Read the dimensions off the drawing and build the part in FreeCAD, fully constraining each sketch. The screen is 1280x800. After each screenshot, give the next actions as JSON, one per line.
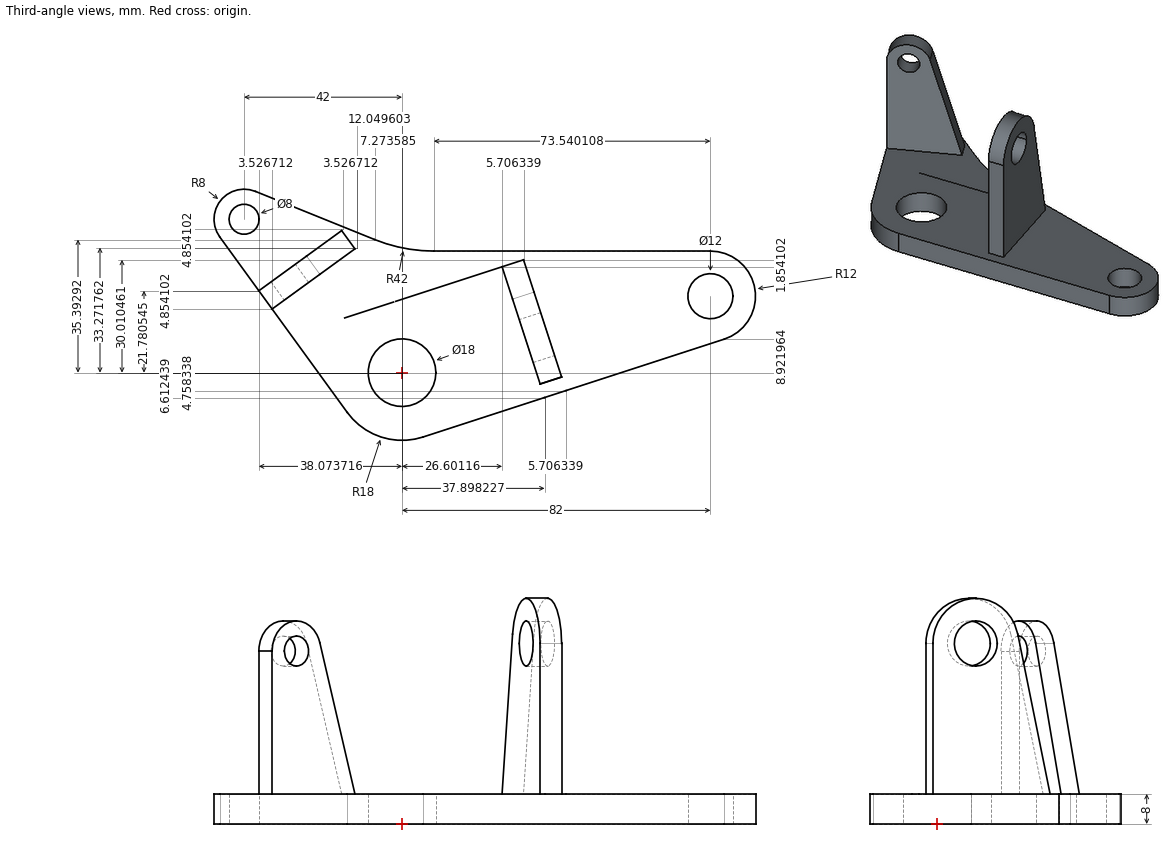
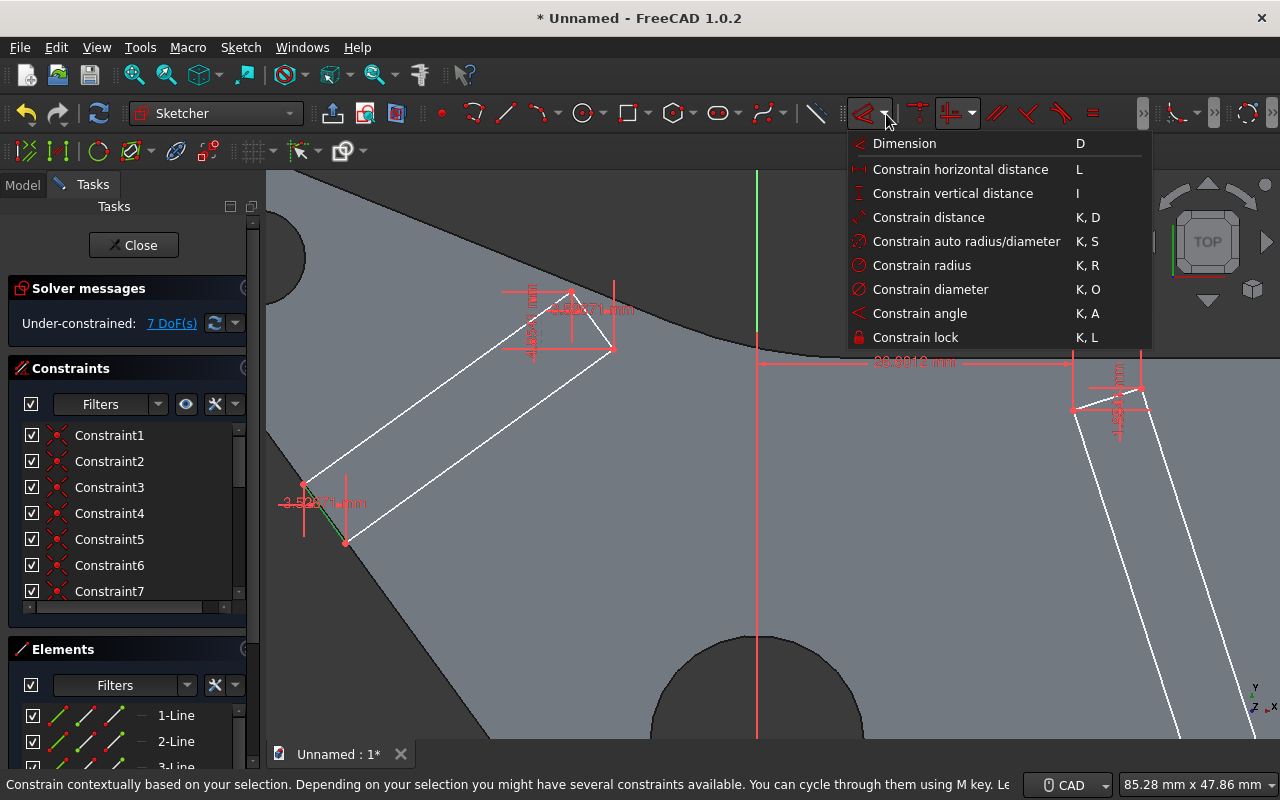
{"action": "left_click", "coordinate": [1000, 193]}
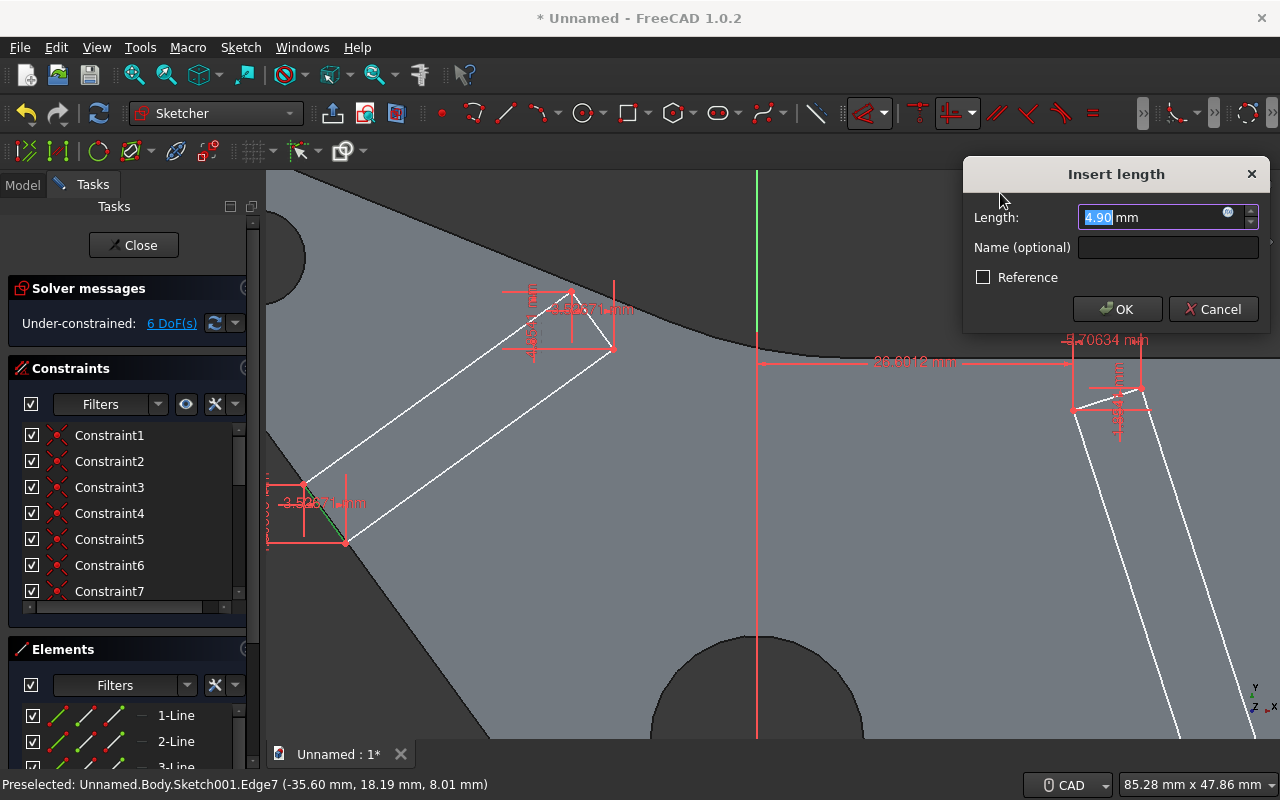
{"action": "type", "text": "4.854102"}
{"action": "key", "text": "Return"}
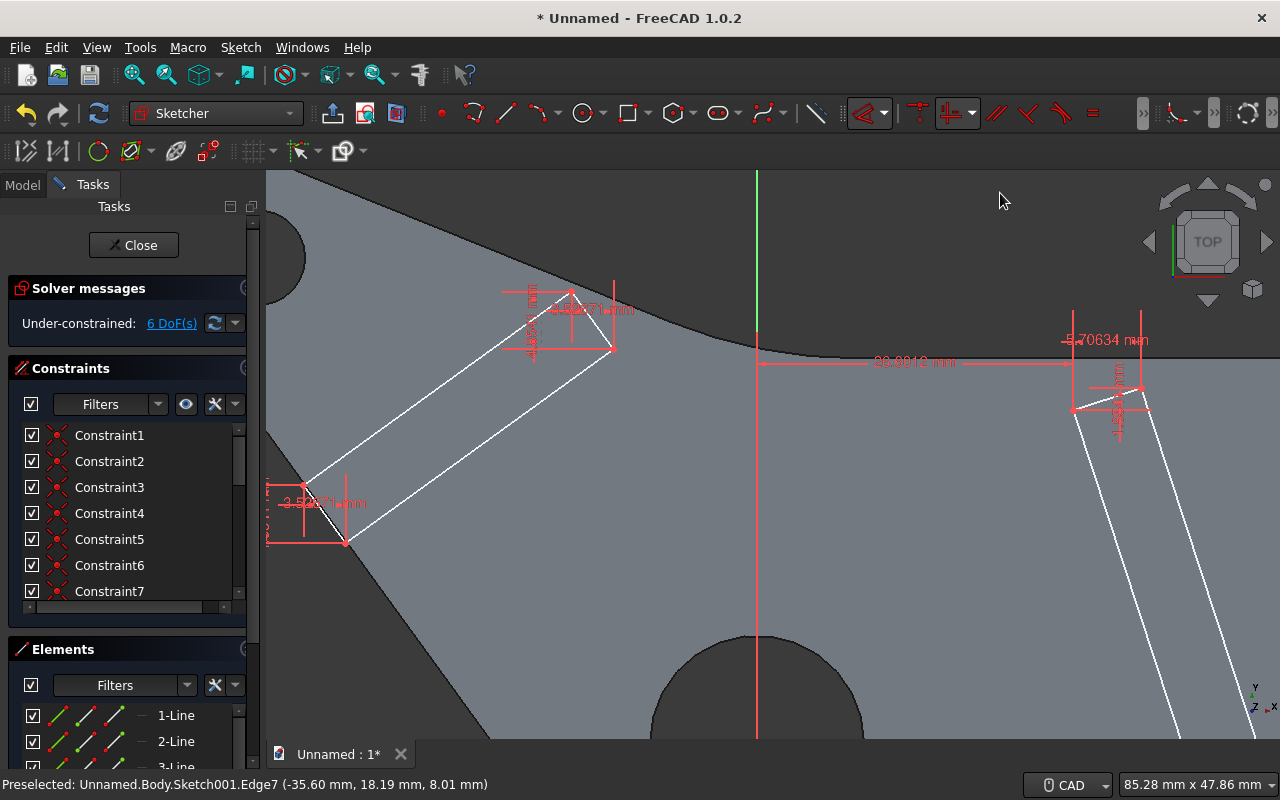
{"action": "scroll", "coordinate": [601, 332], "scroll_direction": "down", "scroll_amount": 3}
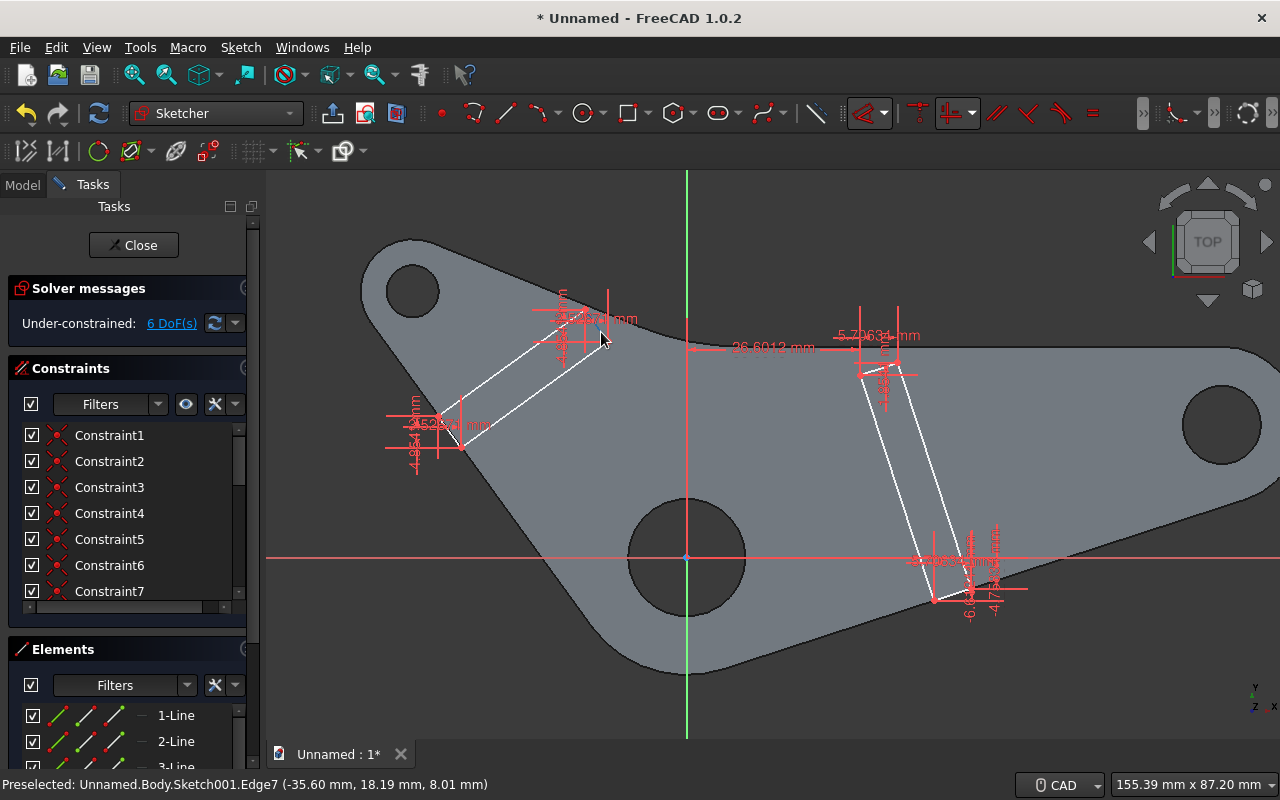
{"action": "left_click", "coordinate": [934, 601]}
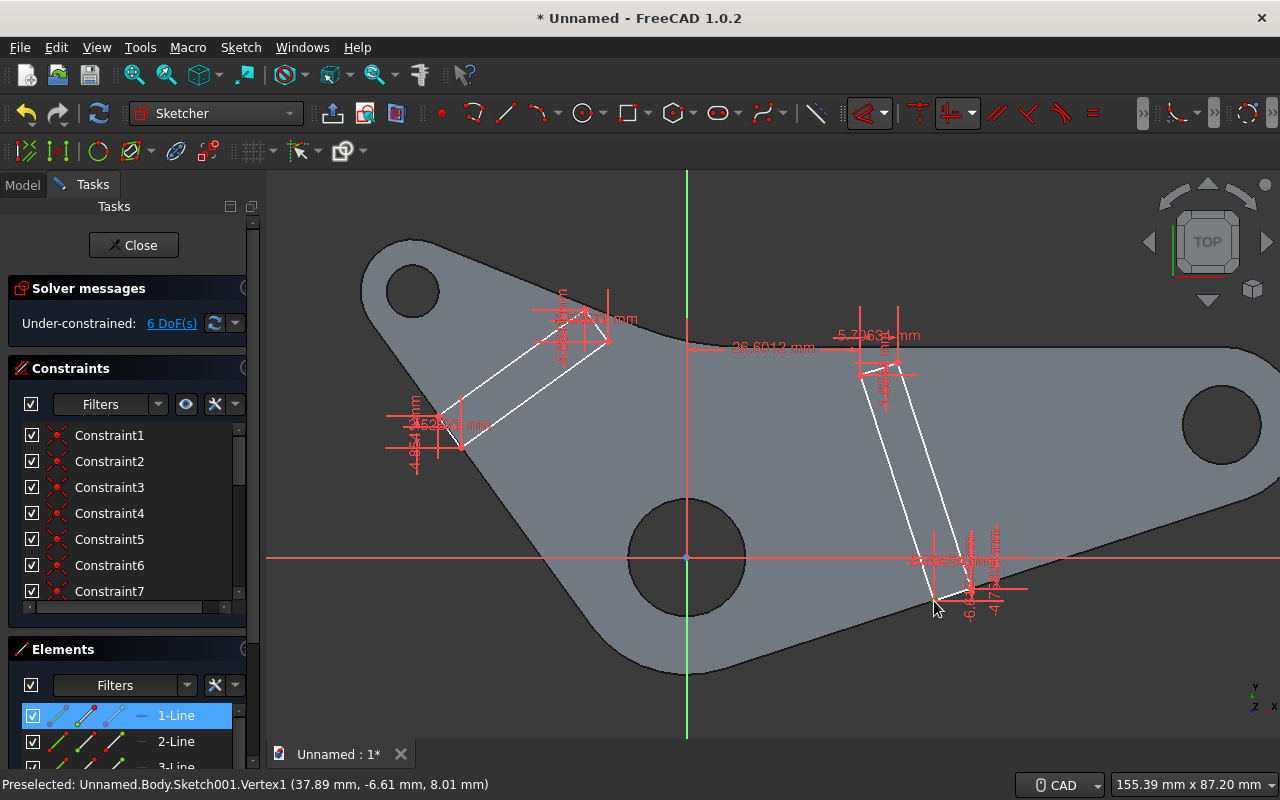
{"action": "key", "text": "l"}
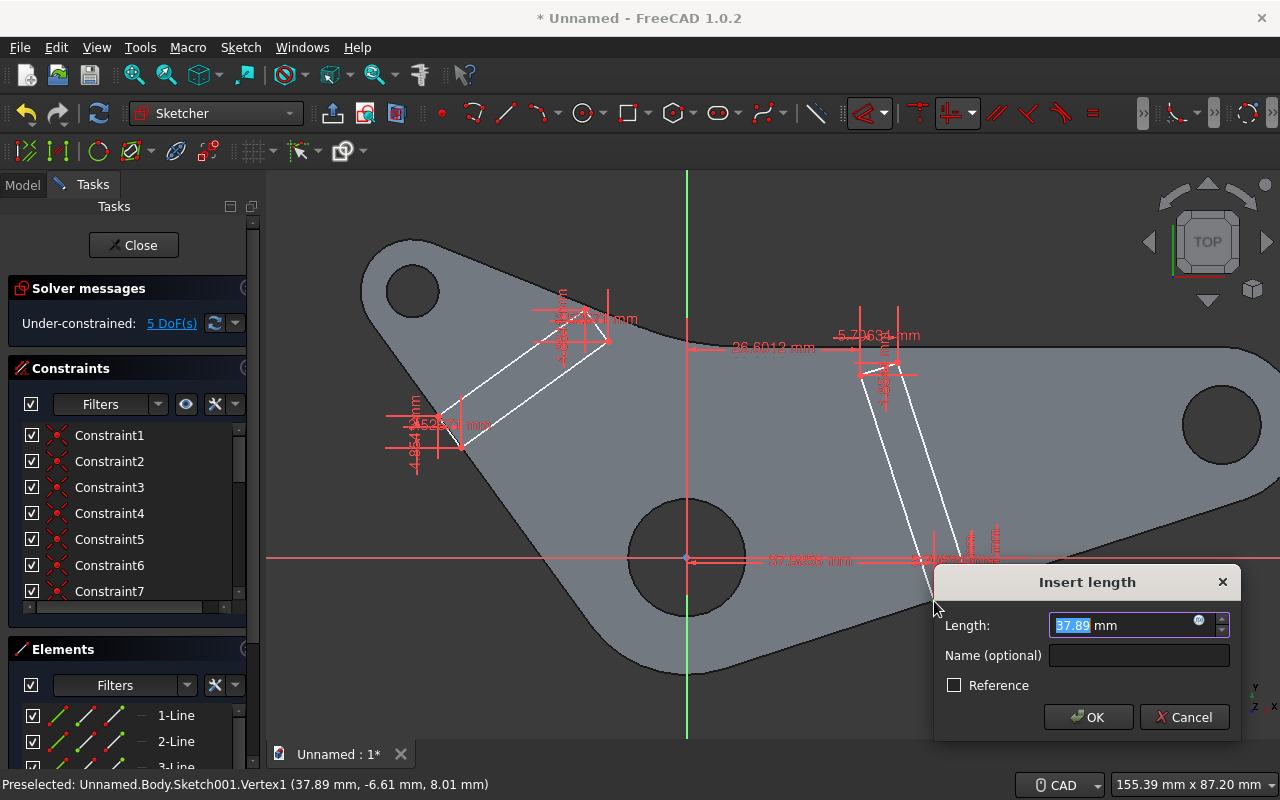
{"action": "type", "text": "37.898227"}
{"action": "key", "text": "Return"}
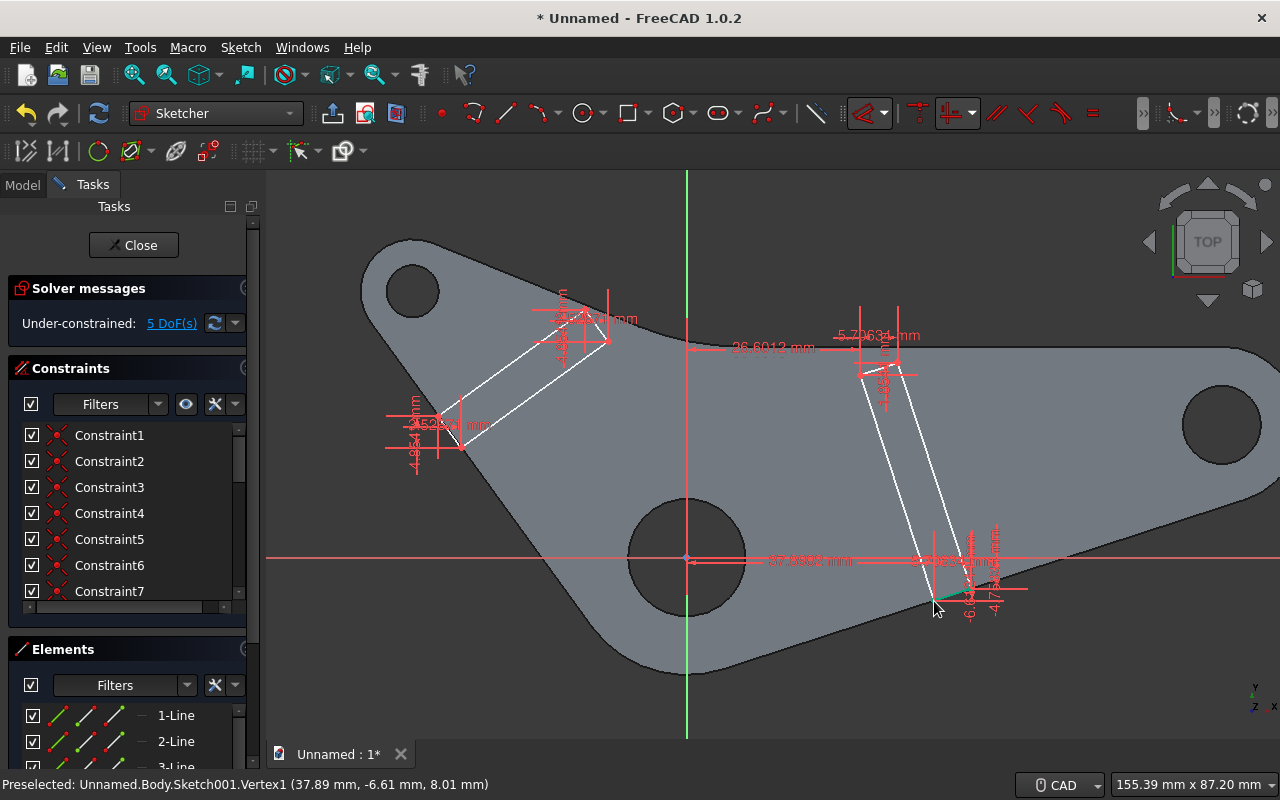
{"action": "left_click", "coordinate": [898, 363]}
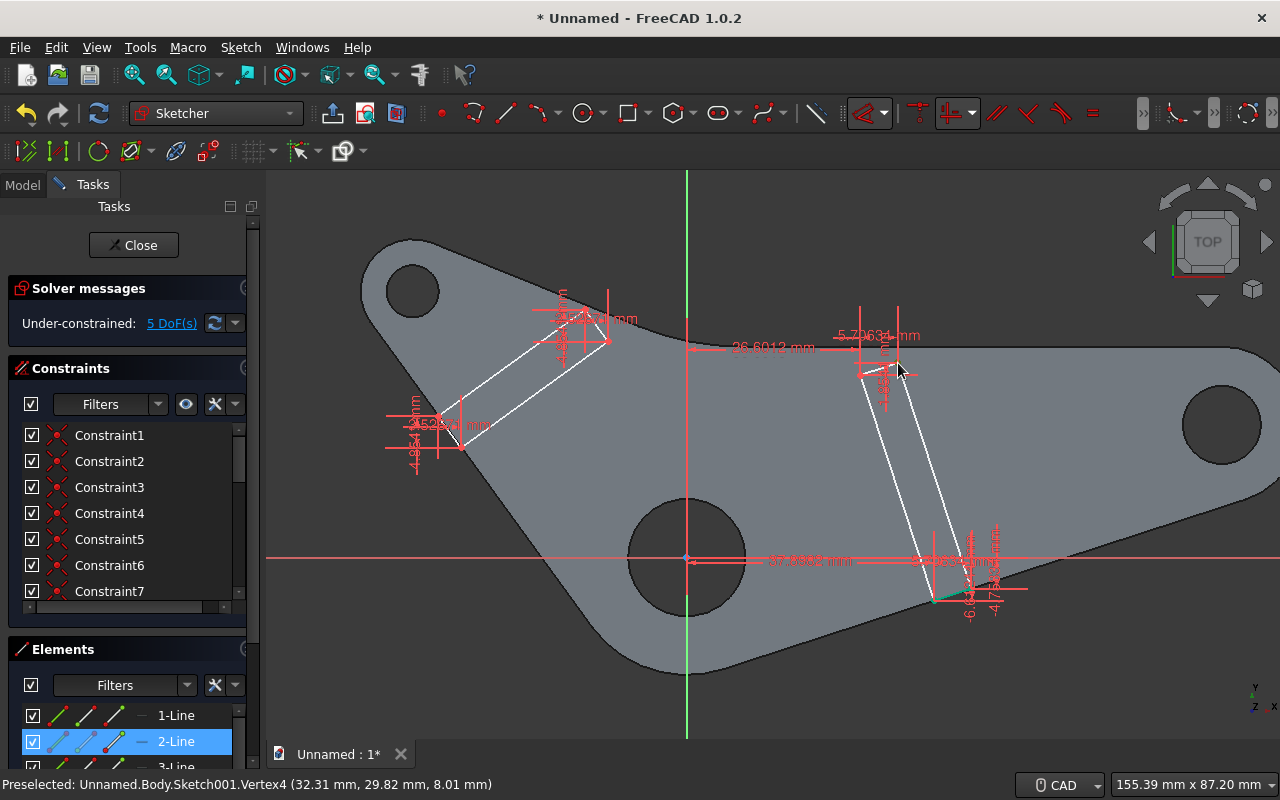
{"action": "key", "text": "i"}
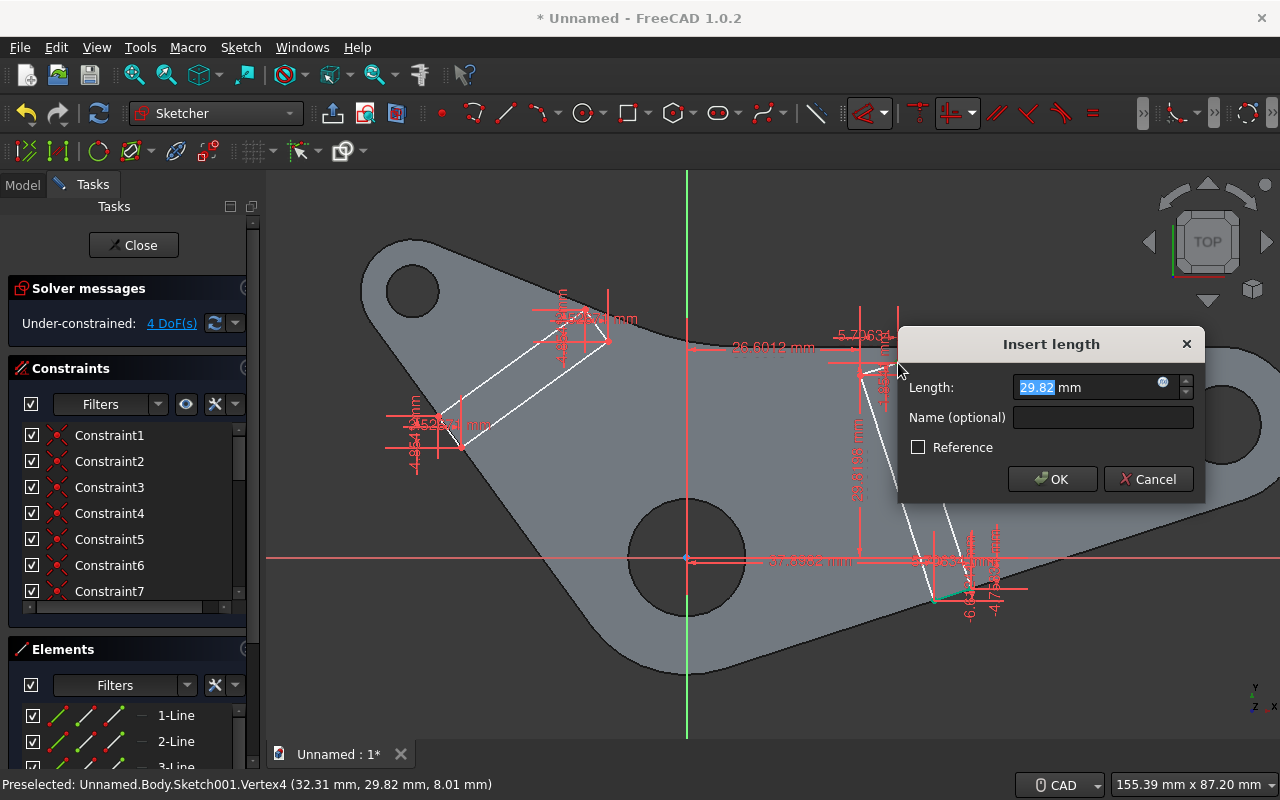
{"action": "type", "text": "30.010461"}
{"action": "key", "text": "Return"}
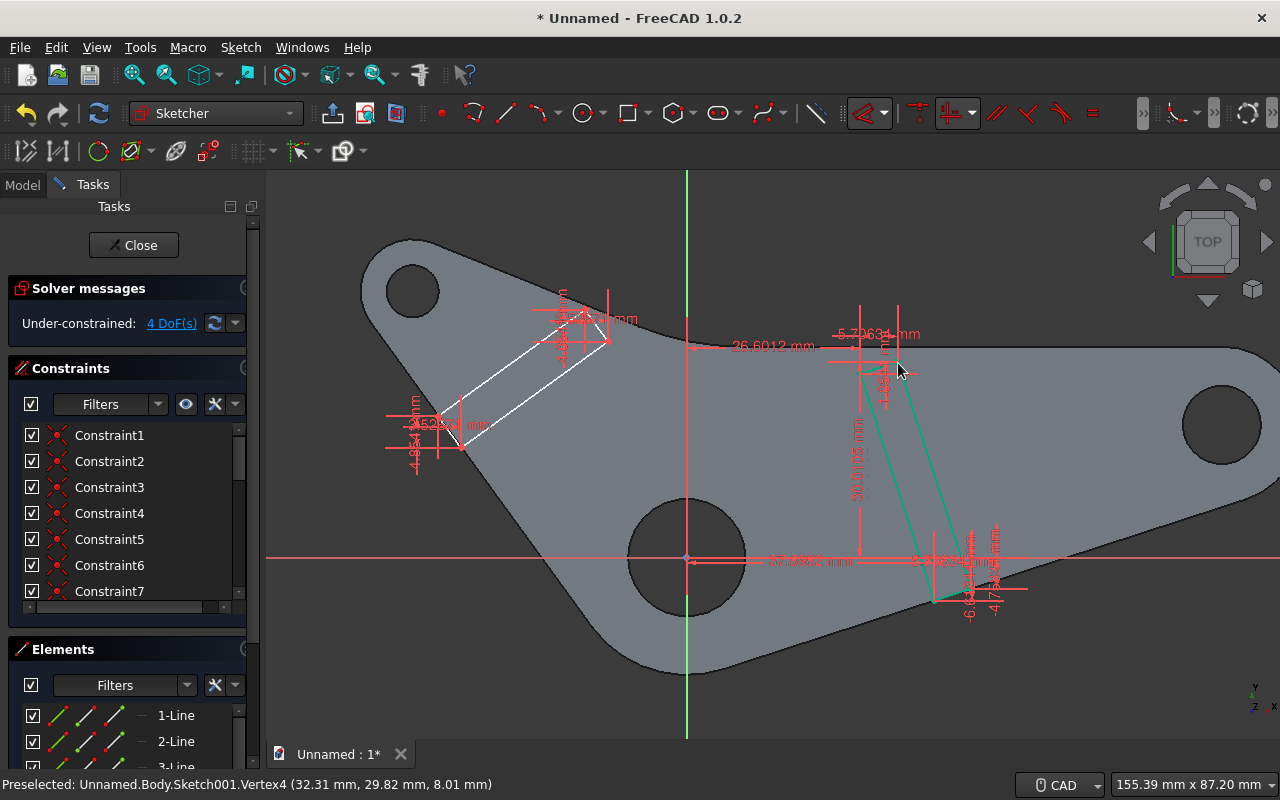
{"action": "left_click", "coordinate": [608, 342]}